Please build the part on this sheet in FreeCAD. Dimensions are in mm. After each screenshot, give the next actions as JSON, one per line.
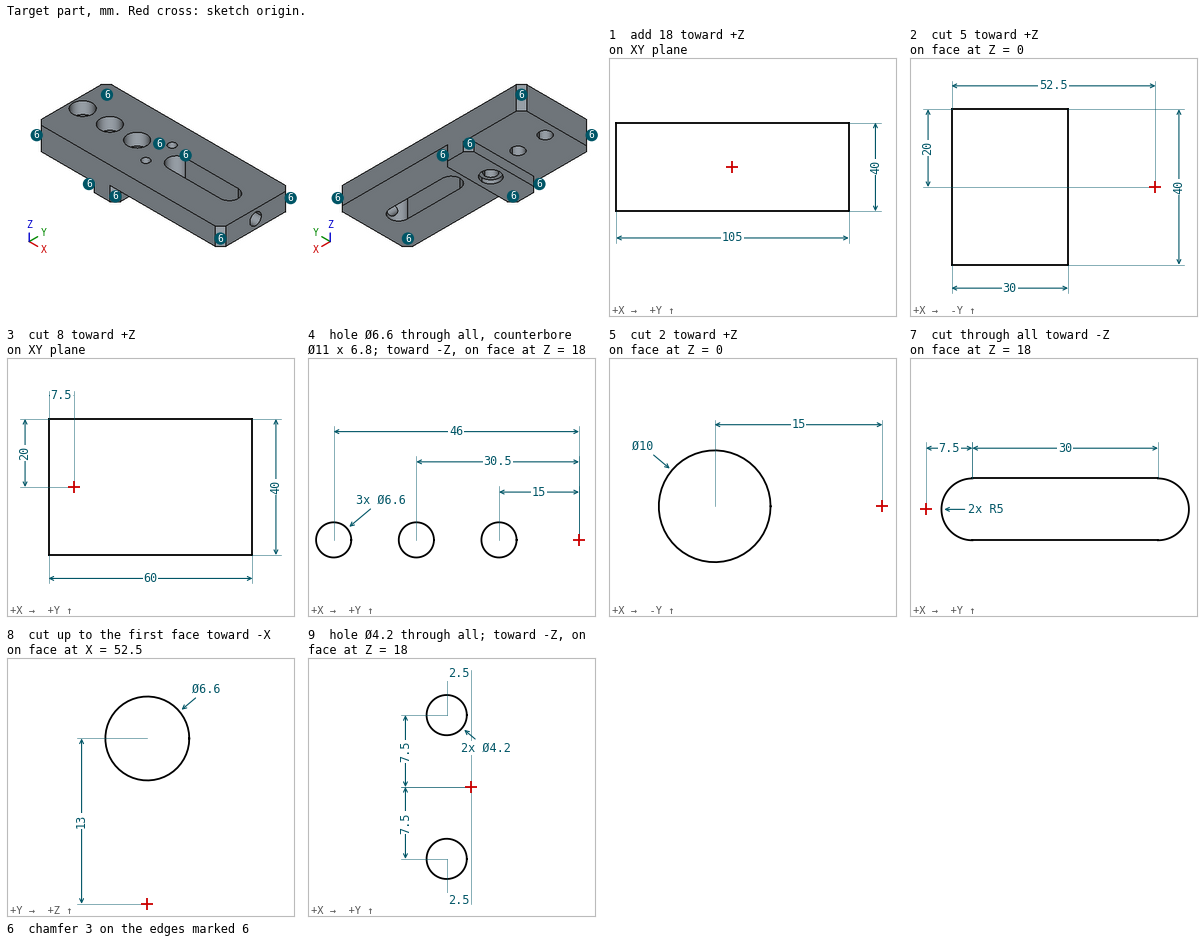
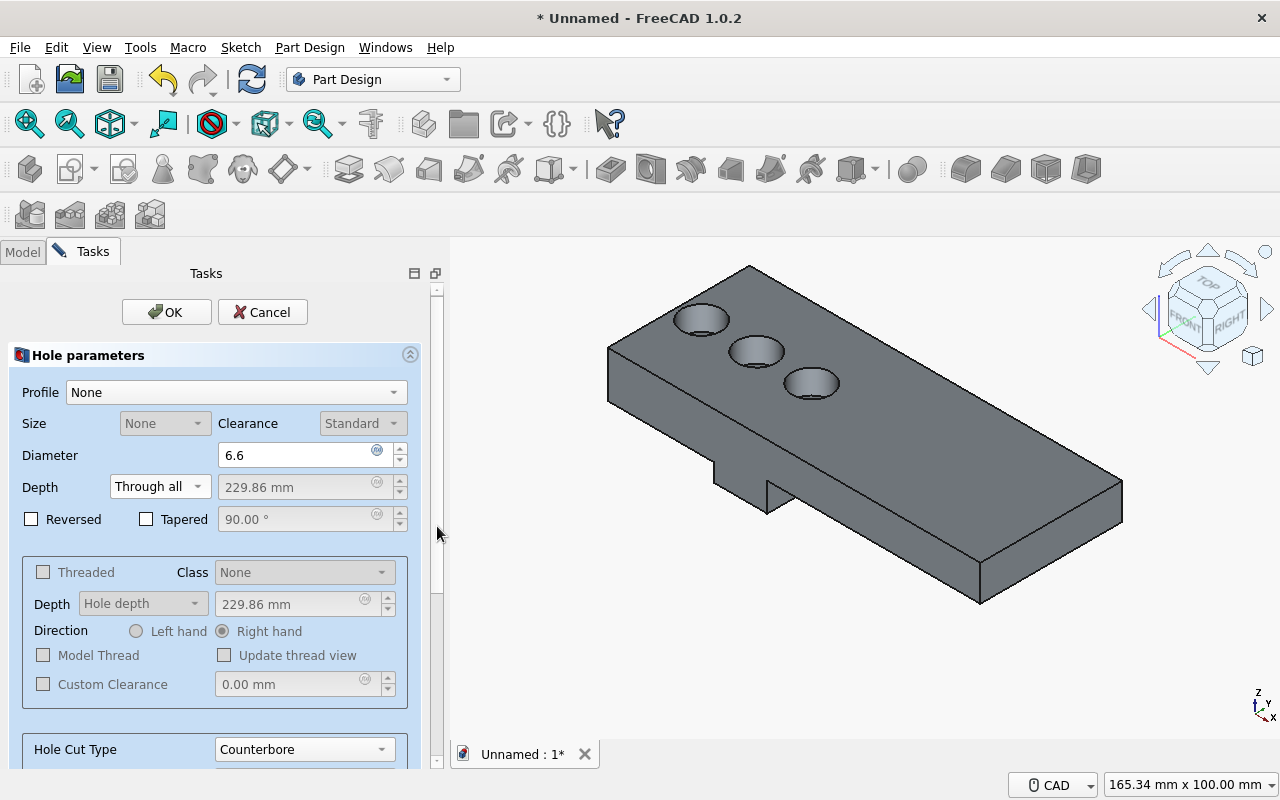
{"action": "left_click", "coordinate": [167, 312]}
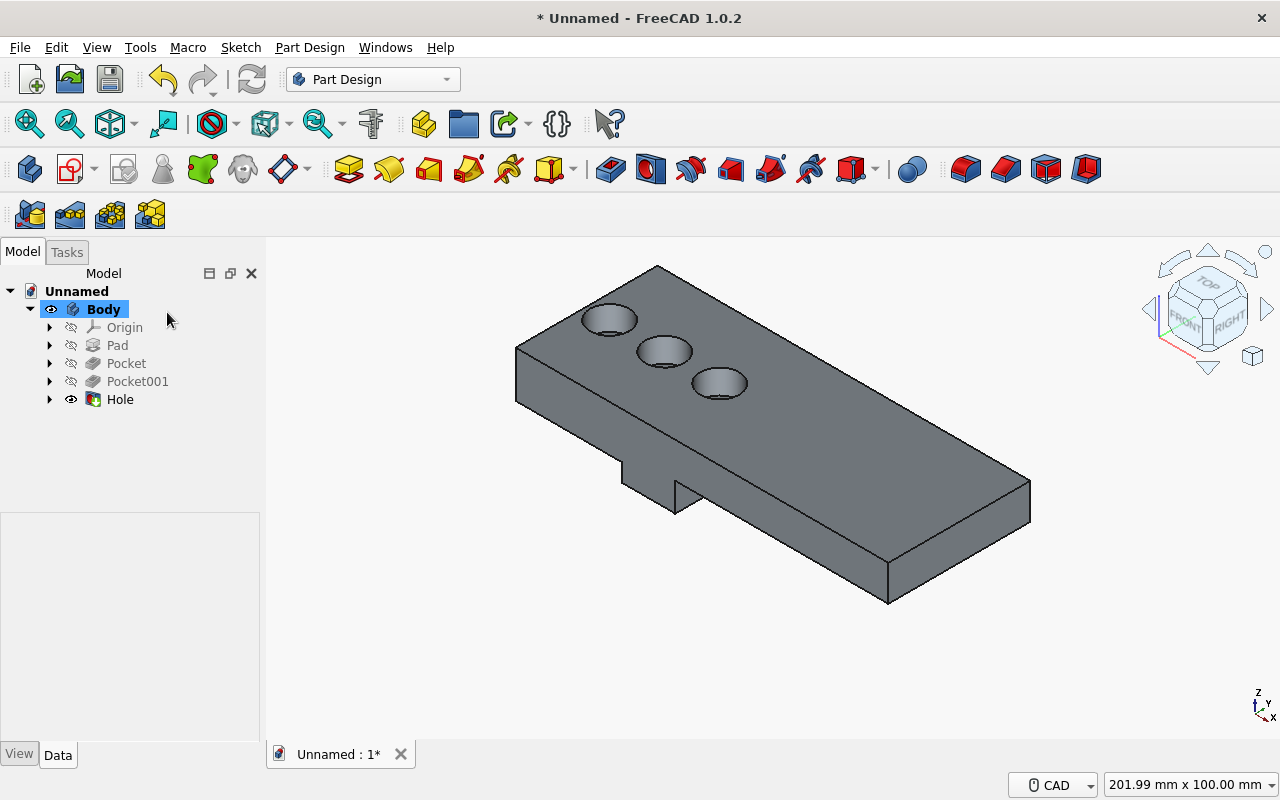
{"action": "key", "text": "5"}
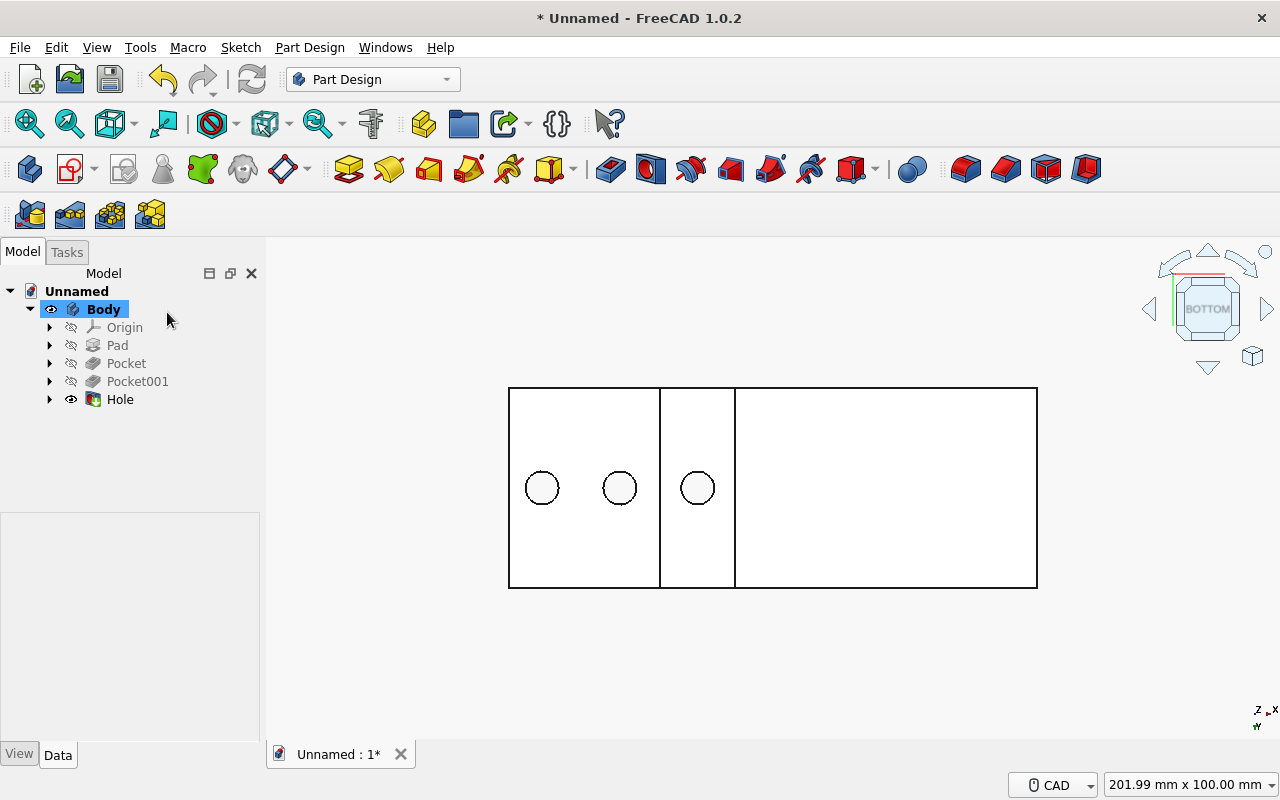
{"action": "left_click", "coordinate": [698, 544]}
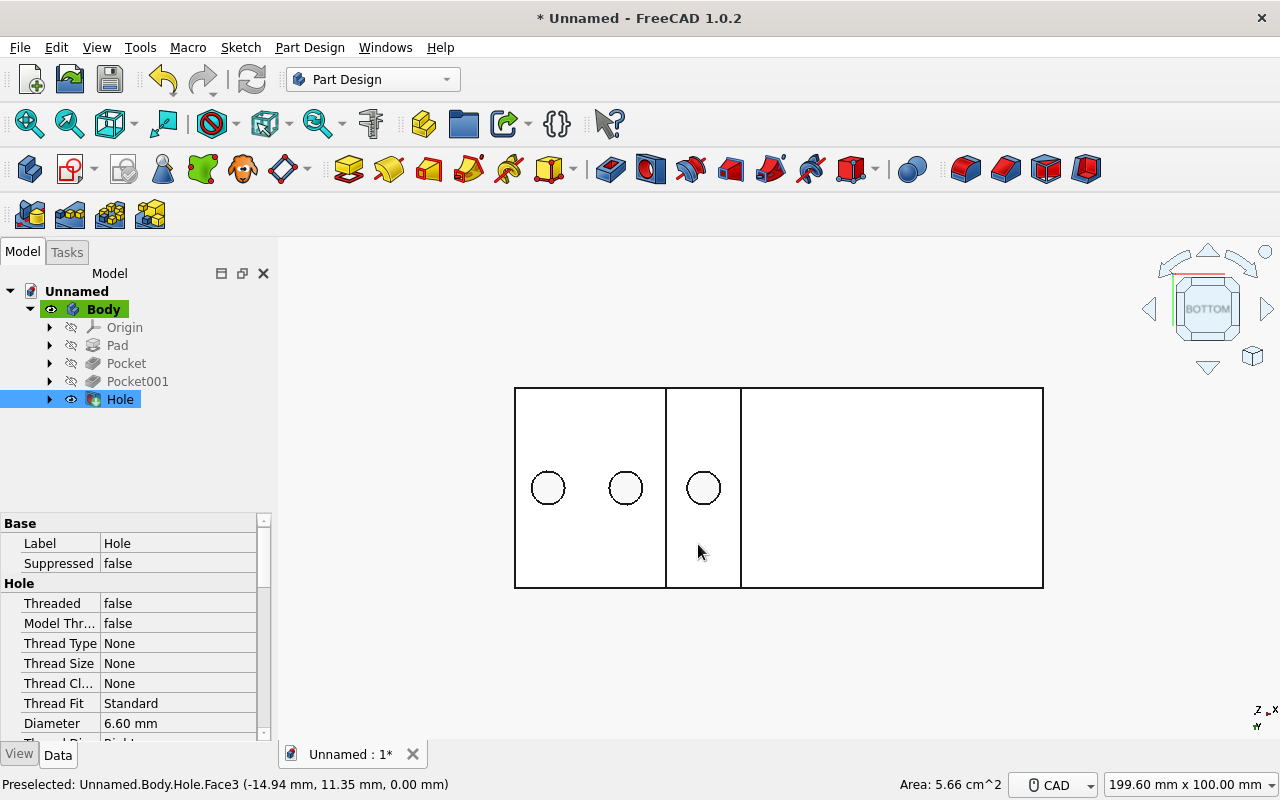
{"action": "left_click", "coordinate": [70, 170]}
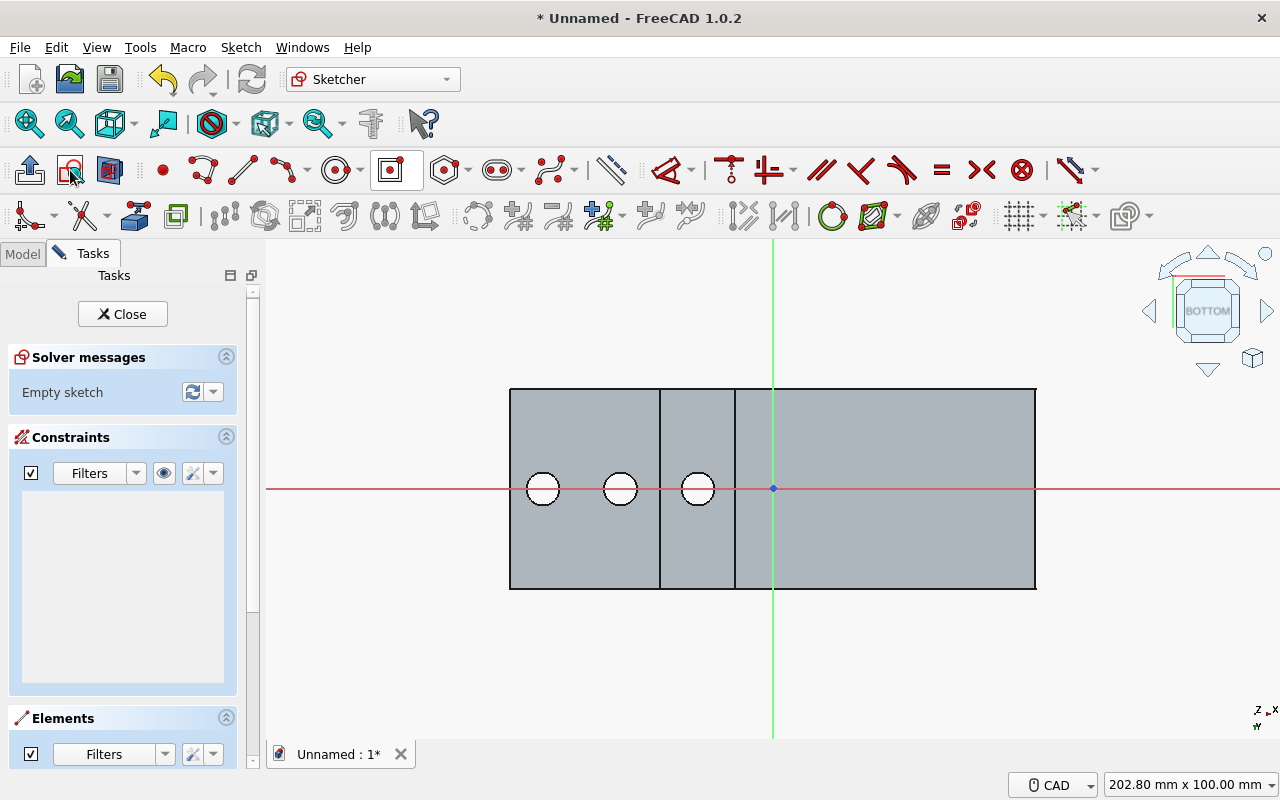
{"action": "scroll", "coordinate": [727, 489], "scroll_direction": "up", "scroll_amount": 9}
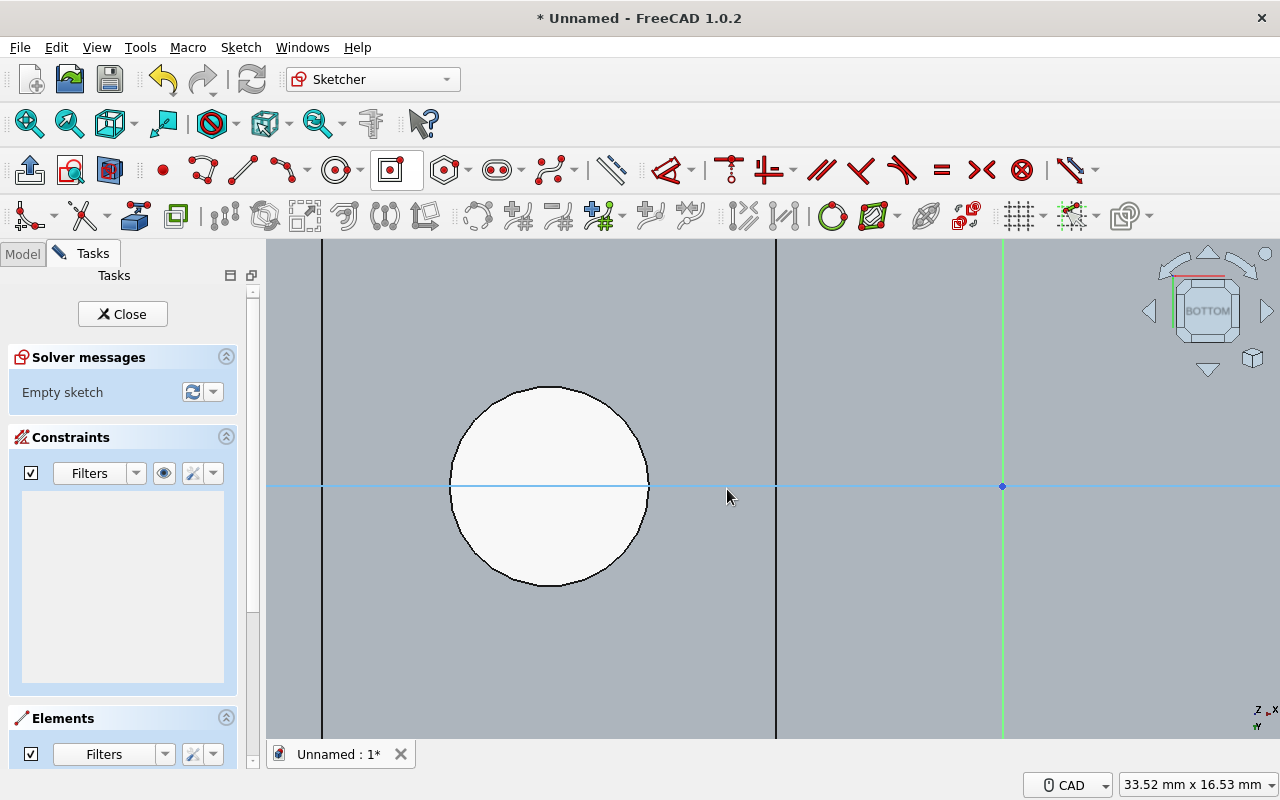
{"action": "left_click", "coordinate": [336, 170]}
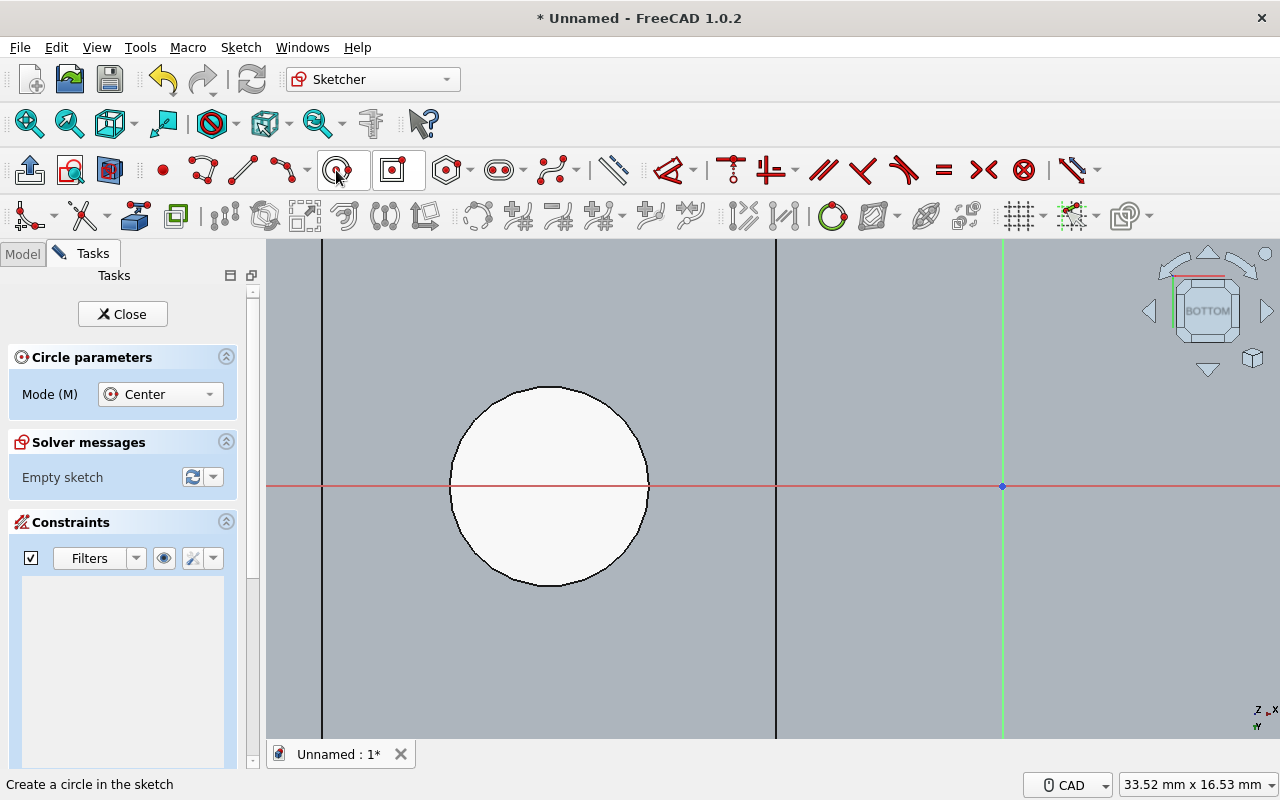
{"action": "left_click", "coordinate": [549, 486]}
{"action": "mouse_move", "coordinate": [656, 380]}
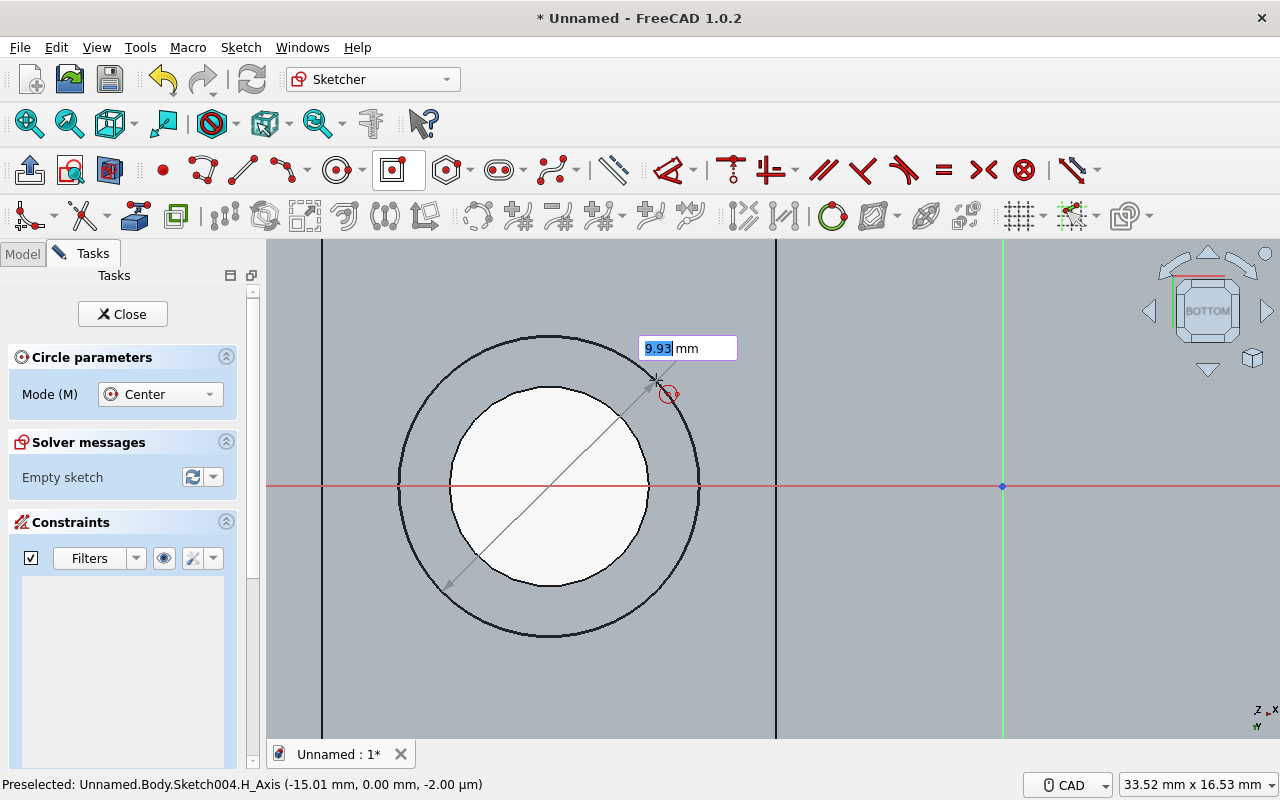
{"action": "type", "text": "10"}
{"action": "key", "text": "Return"}
{"action": "key", "text": "Escape"}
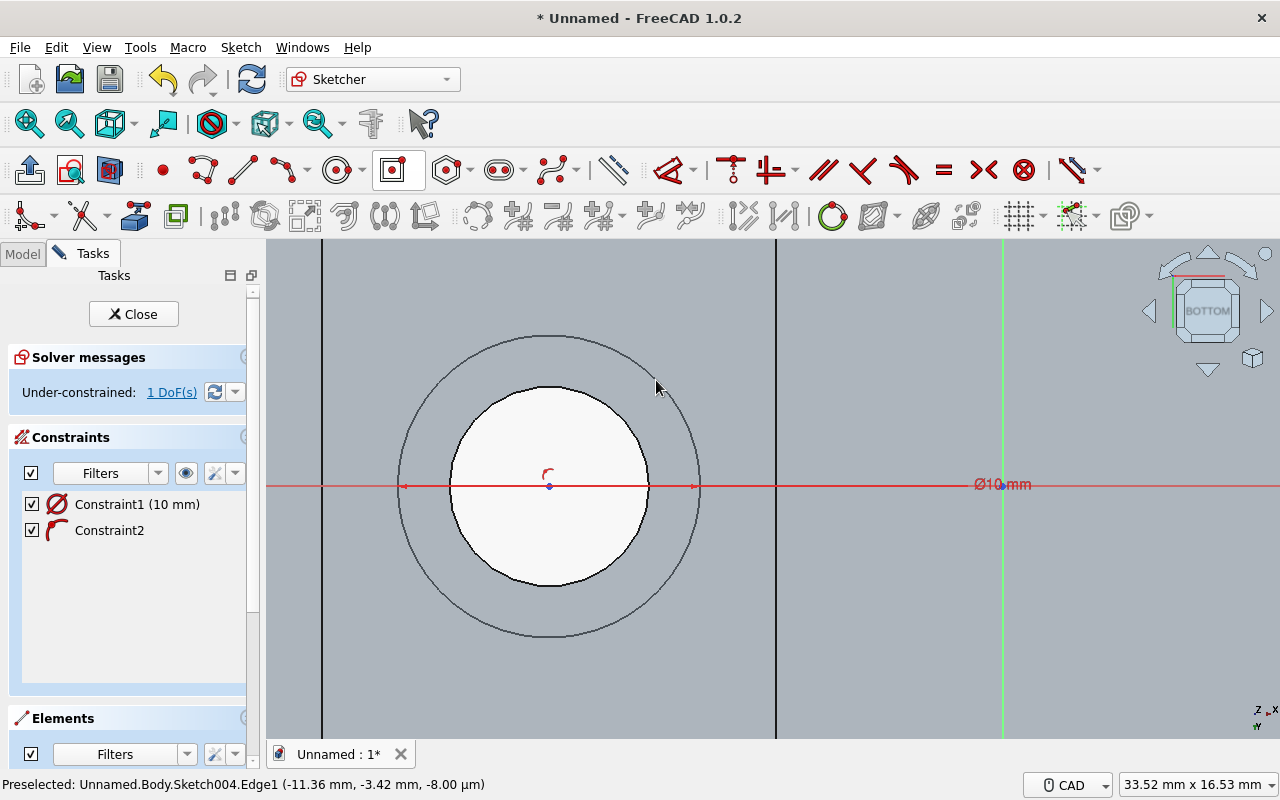
{"action": "left_click", "coordinate": [668, 170]}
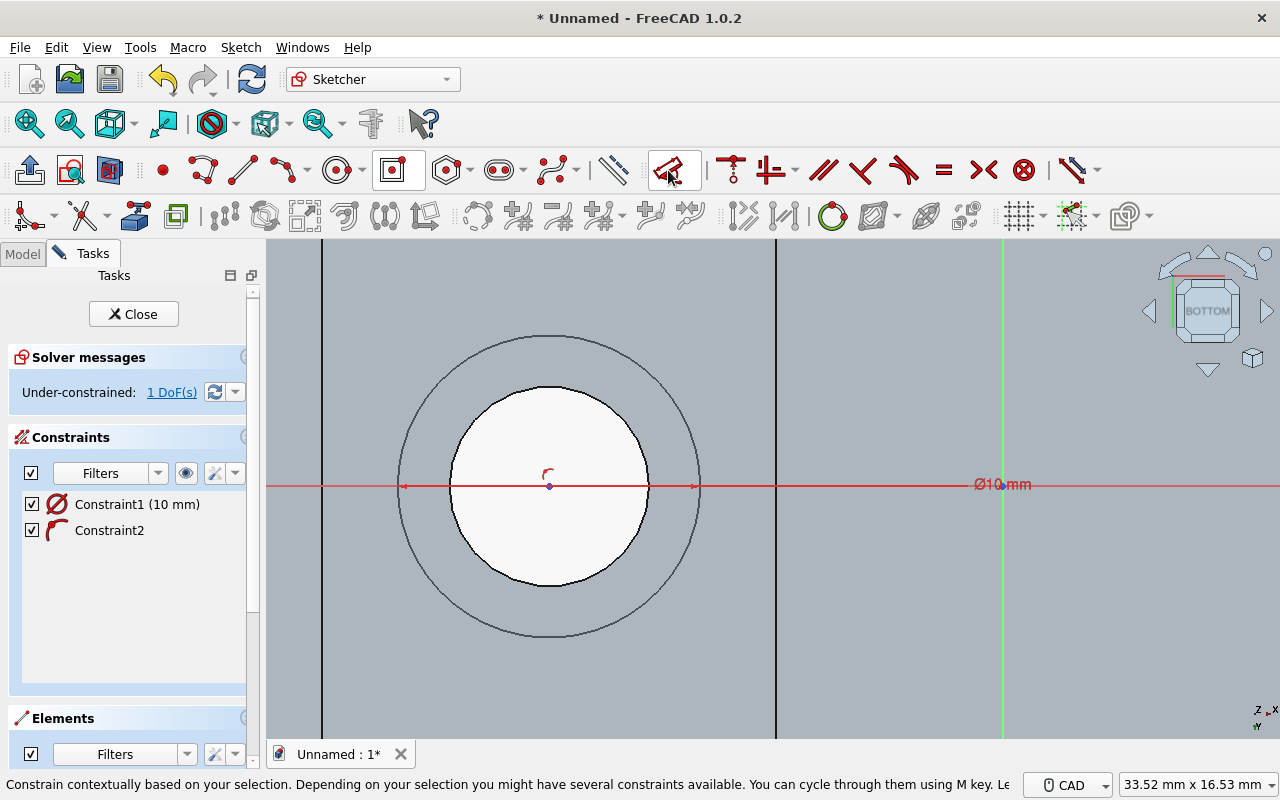
{"action": "left_click", "coordinate": [549, 486]}
{"action": "left_click", "coordinate": [776, 520]}